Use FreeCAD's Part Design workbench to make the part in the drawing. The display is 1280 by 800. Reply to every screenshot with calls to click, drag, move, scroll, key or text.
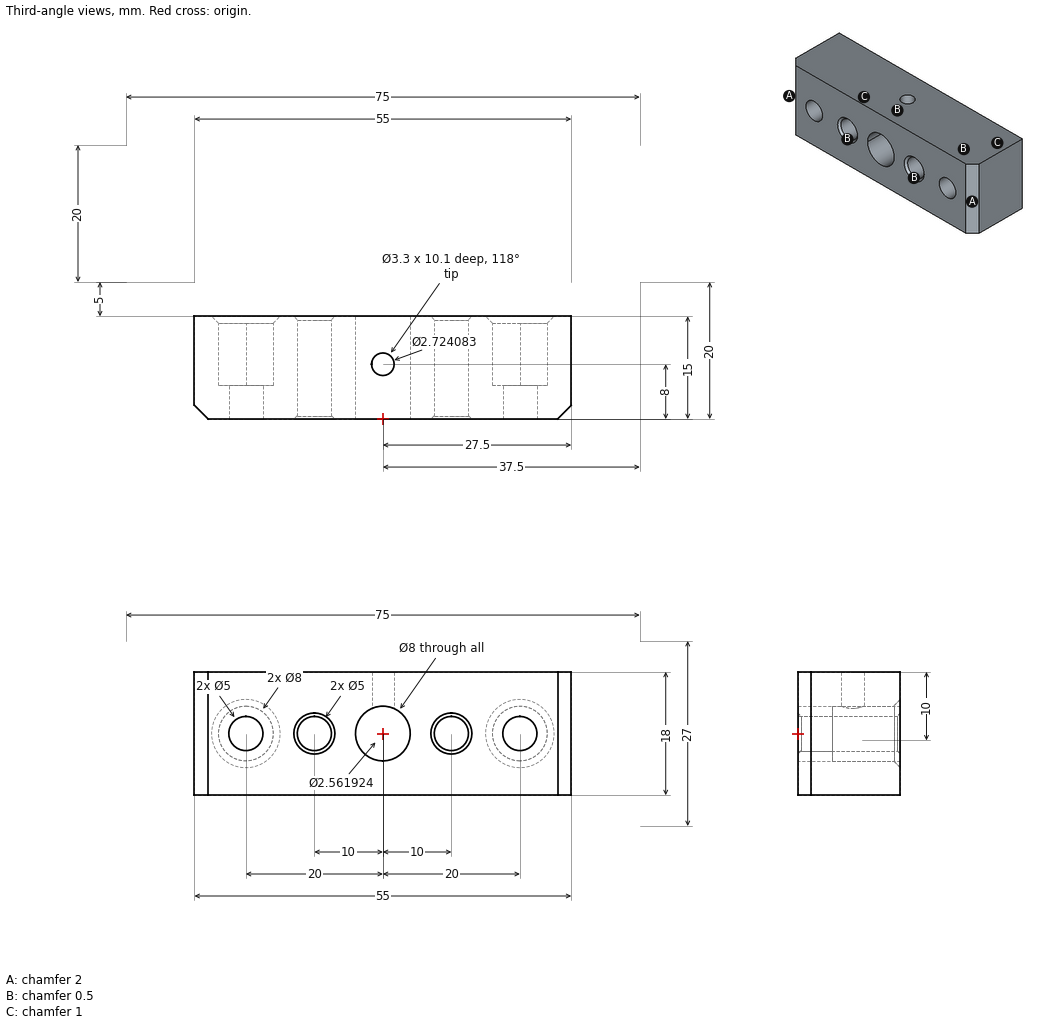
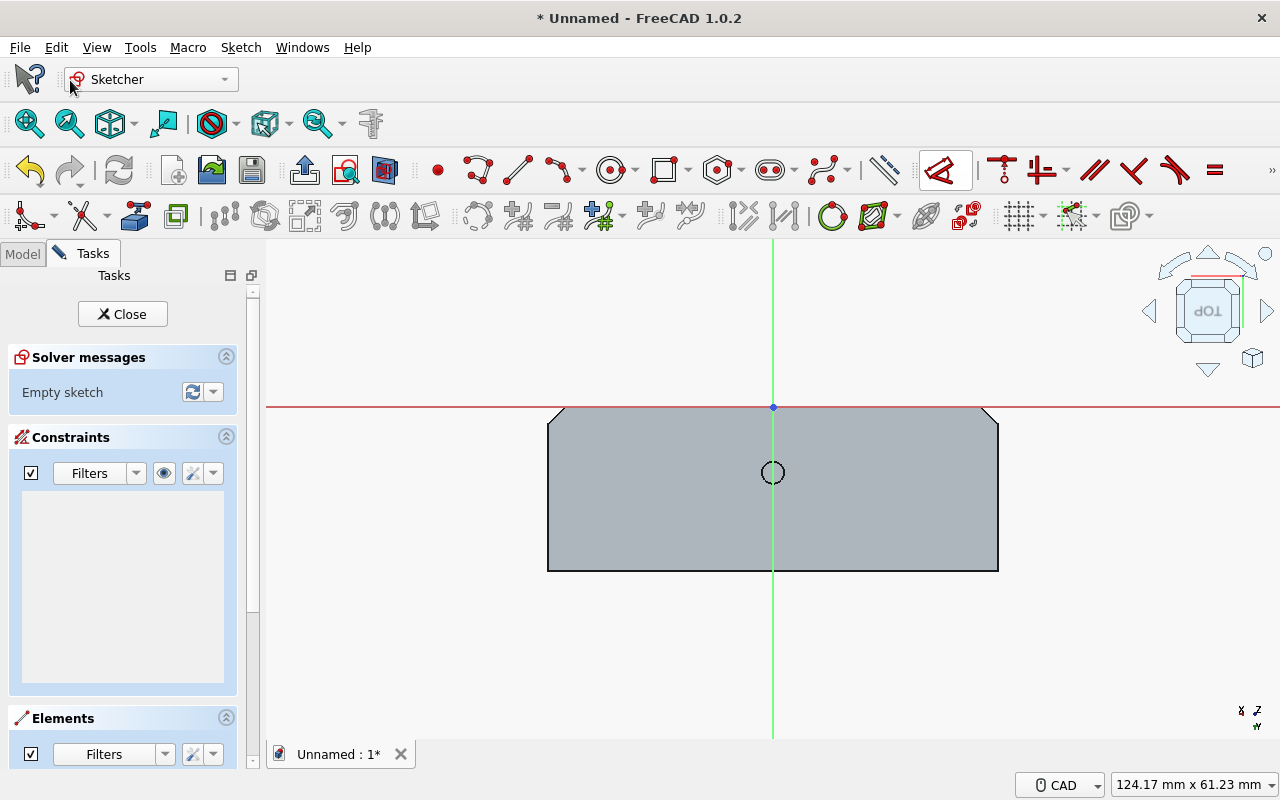
scroll(780, 471, up, 12)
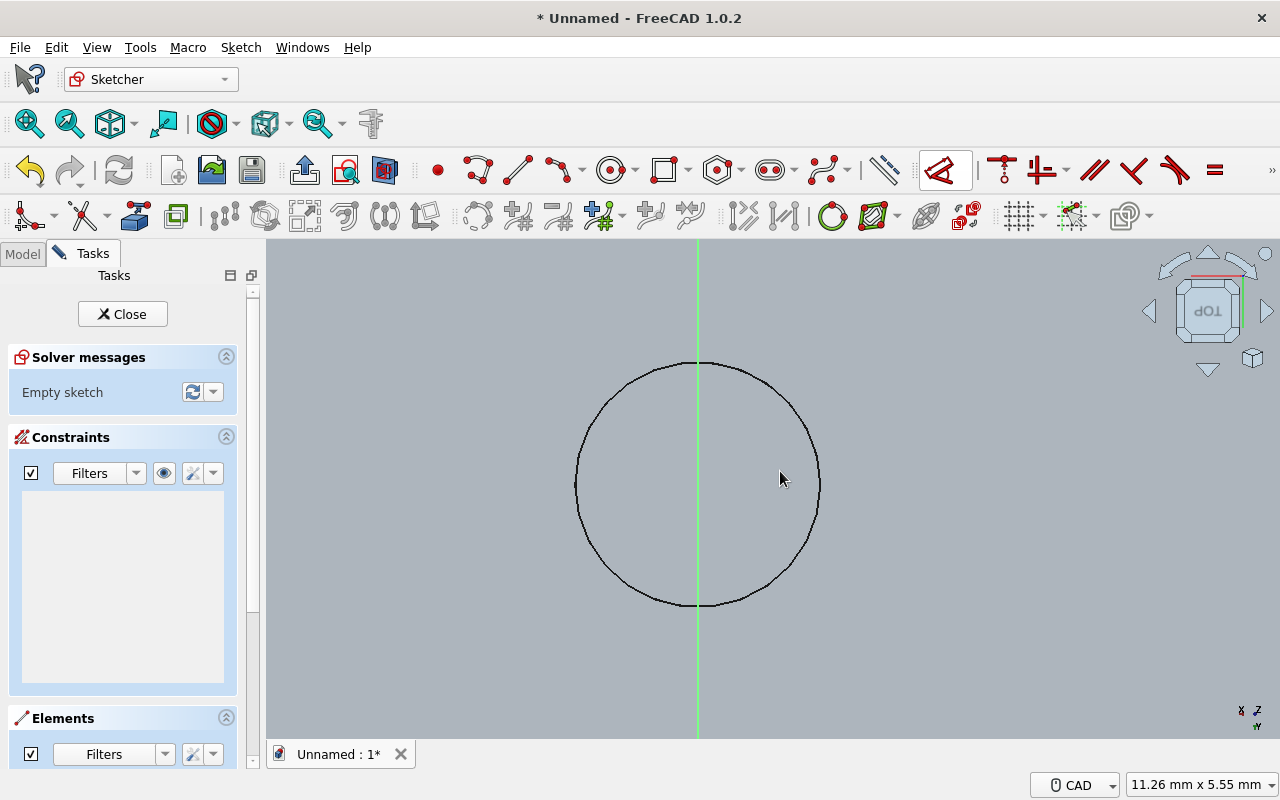
click(612, 170)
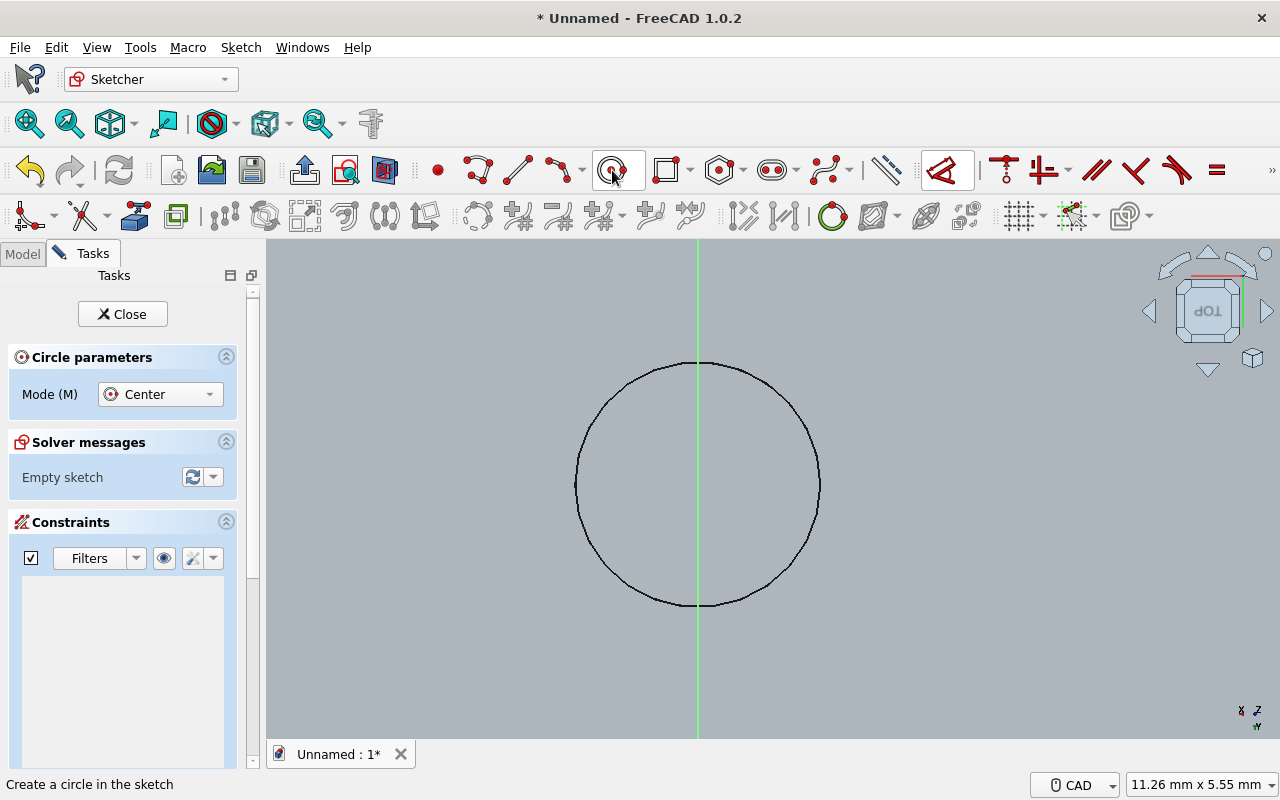
click(698, 485)
move(803, 380)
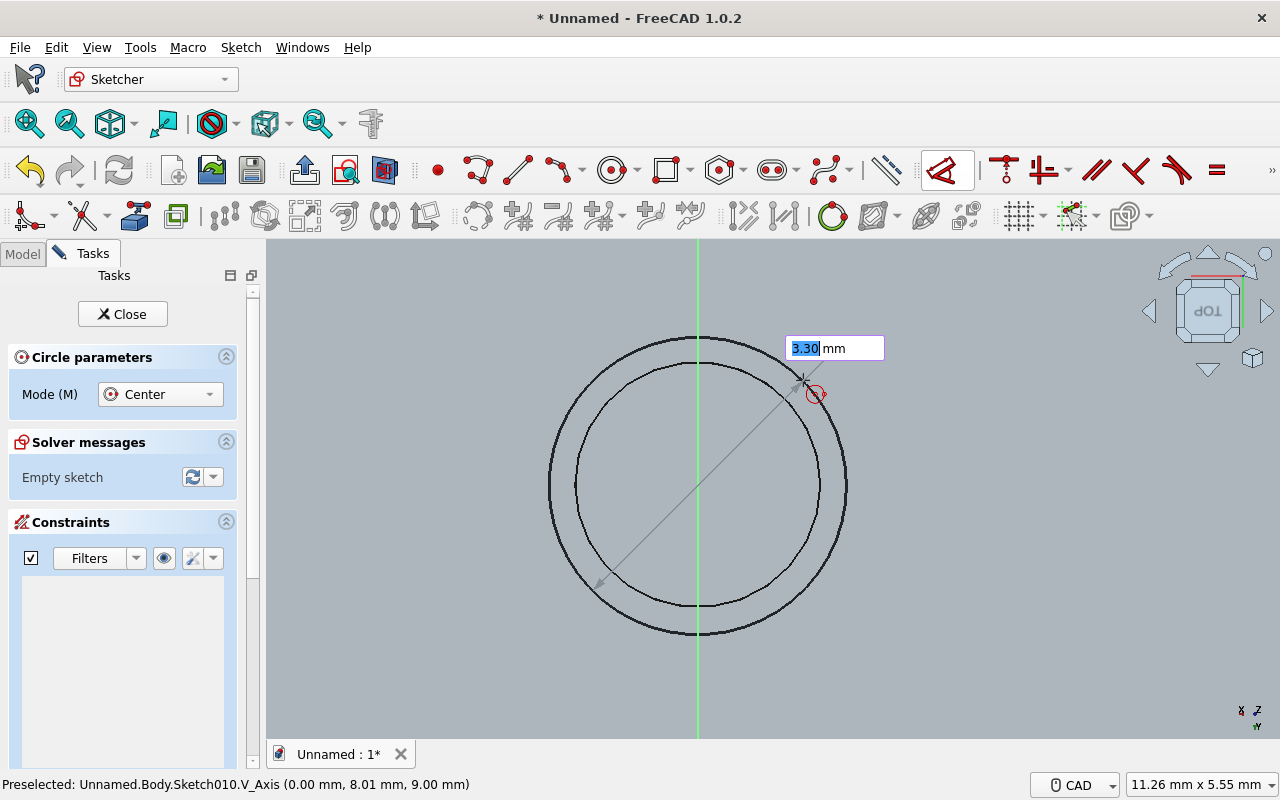
text(3.3)
key(Return)
key(Escape)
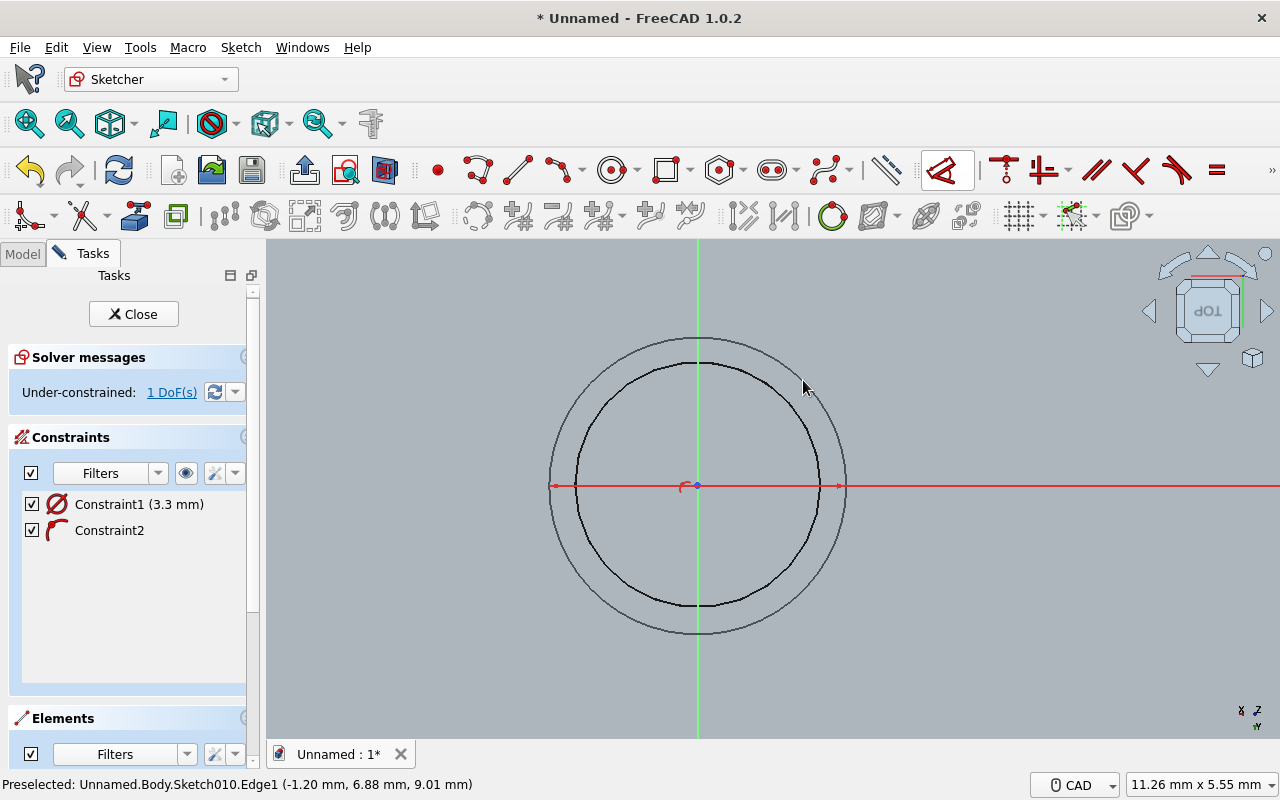
click(698, 486)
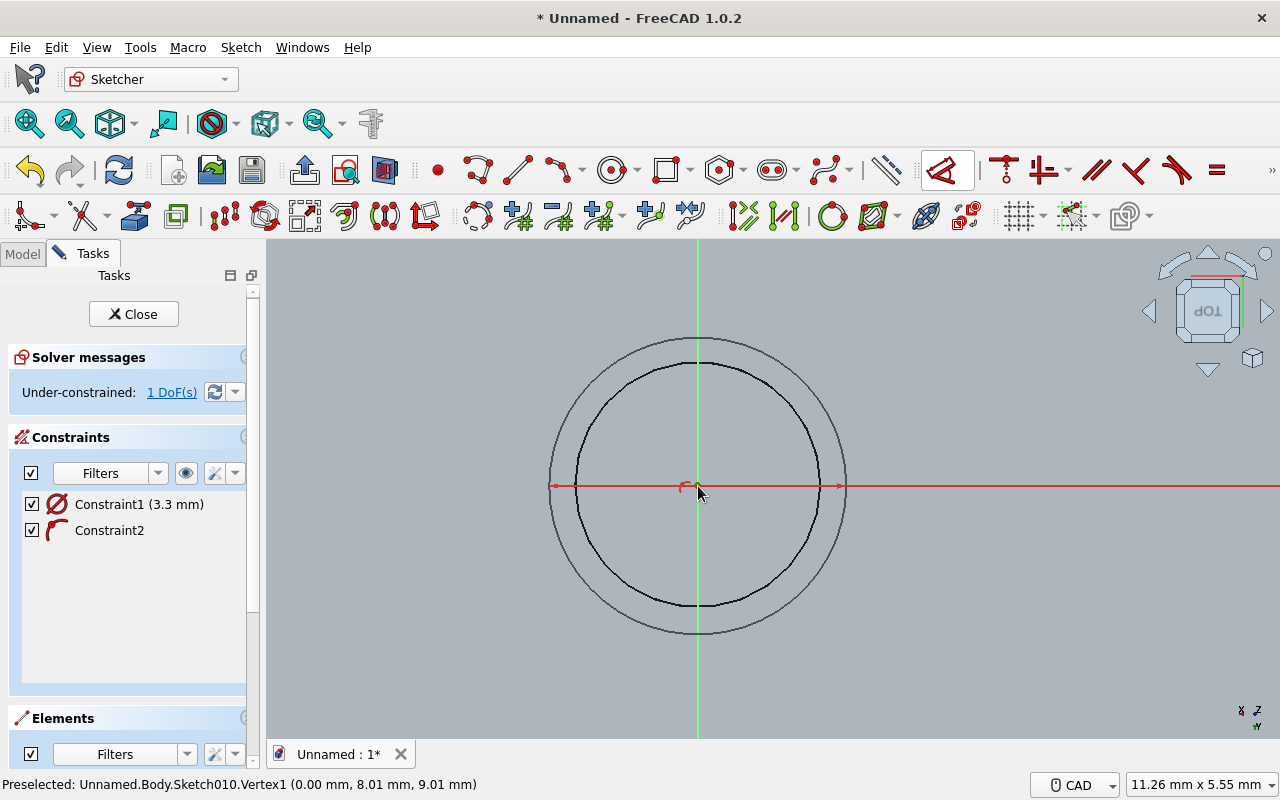
click(968, 170)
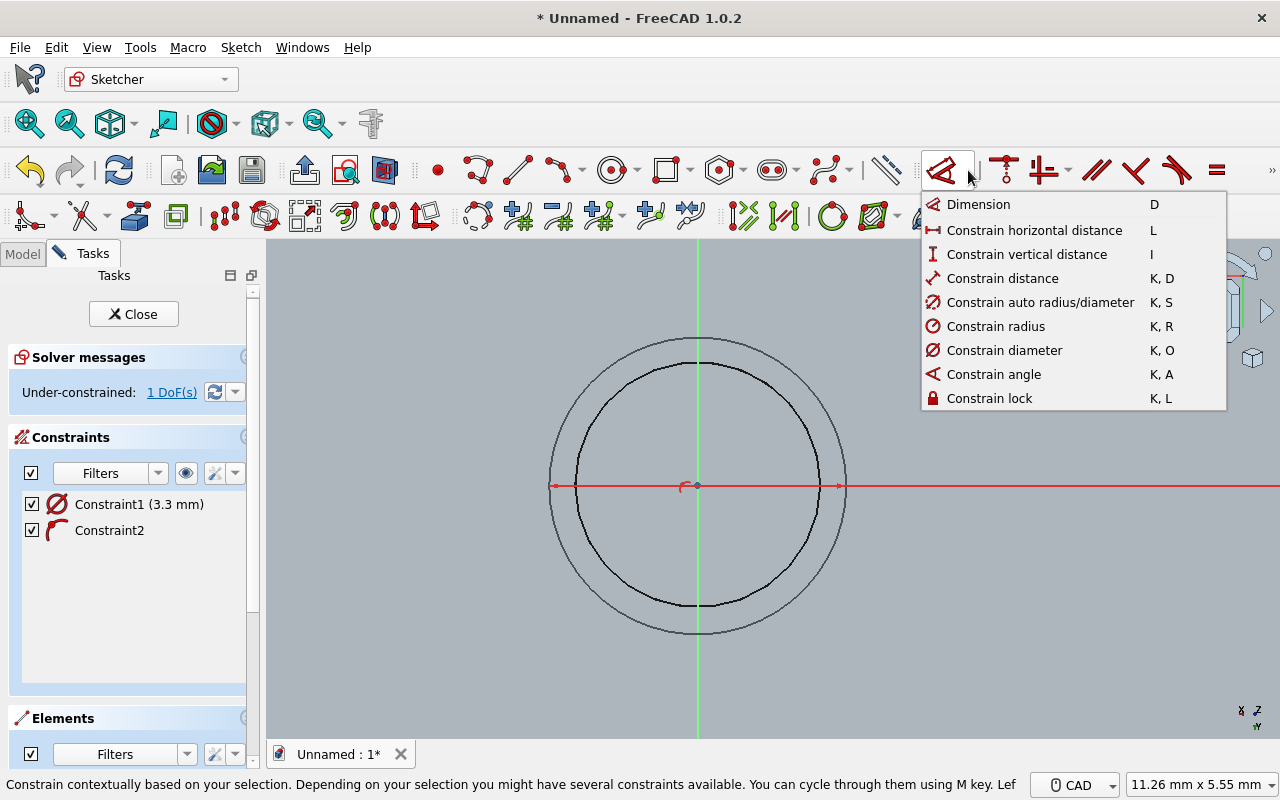
click(1074, 254)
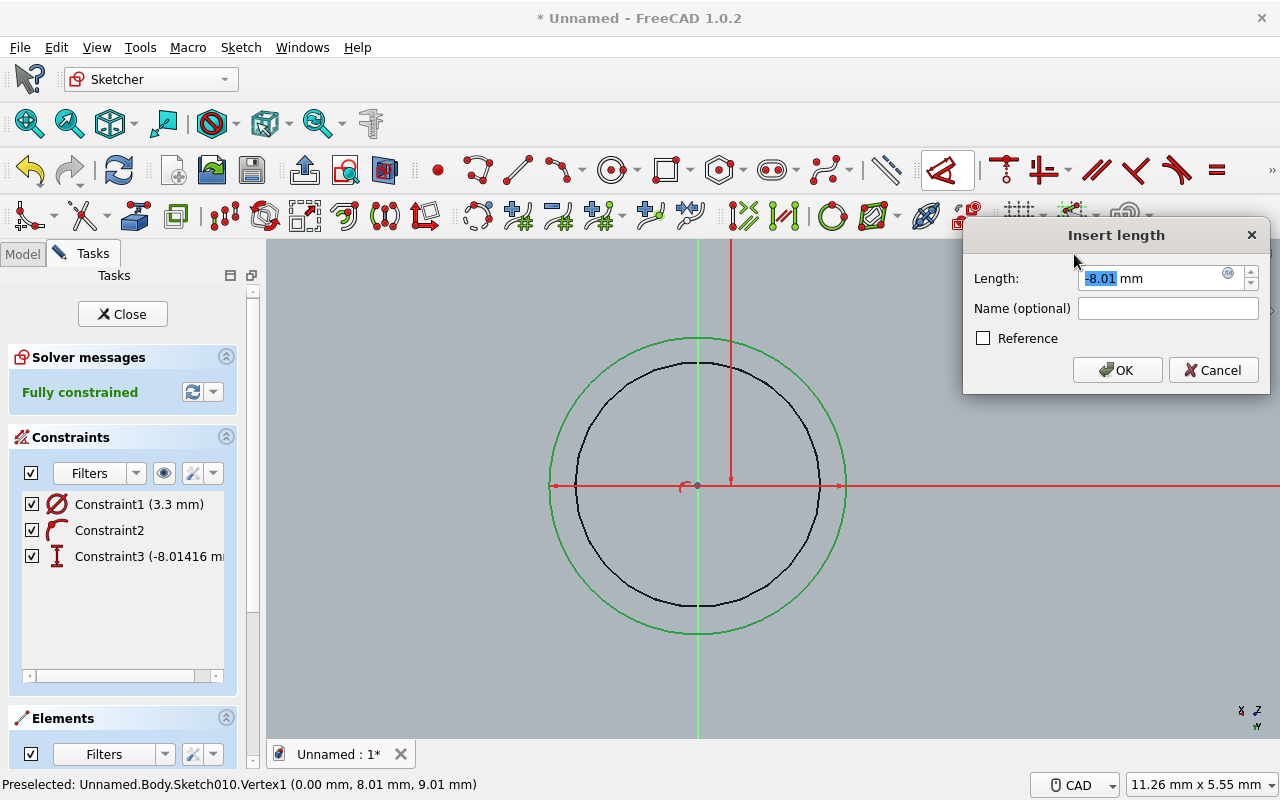
text(-8)
key(Return)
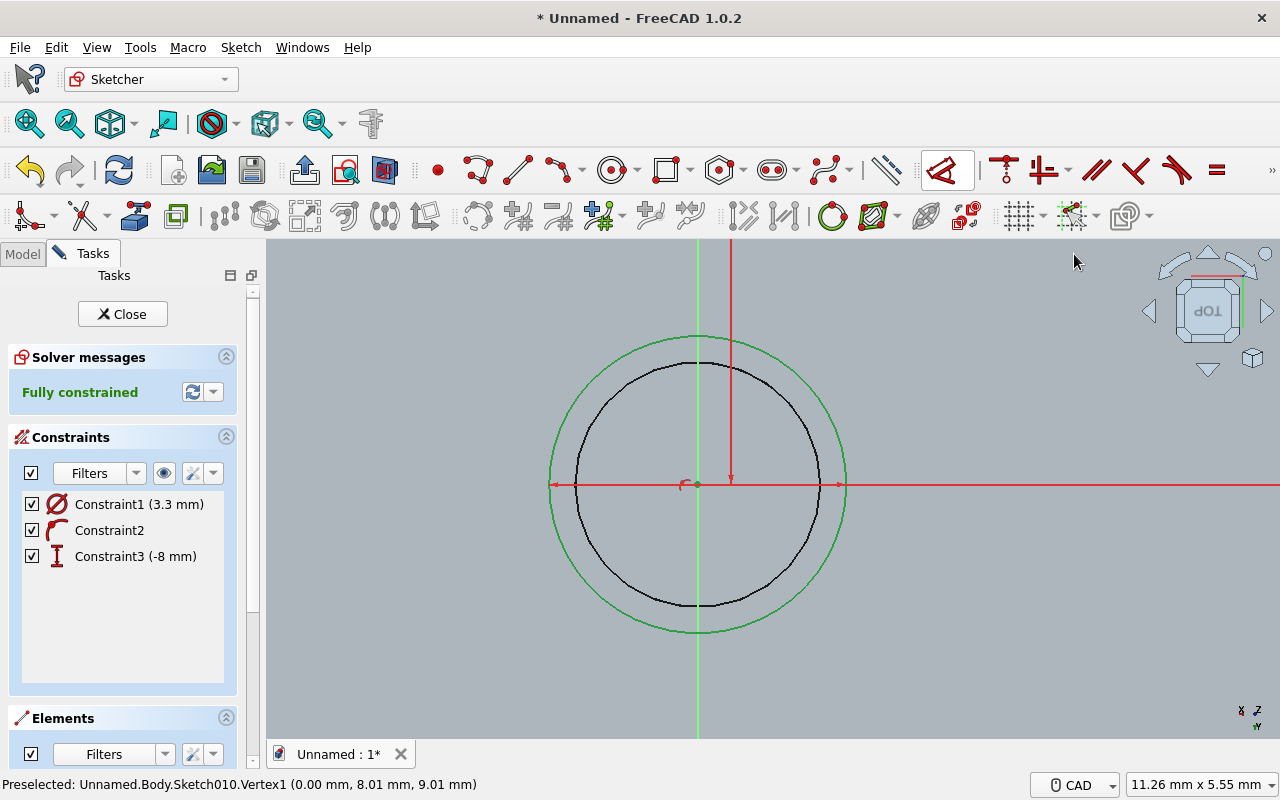
click(123, 314)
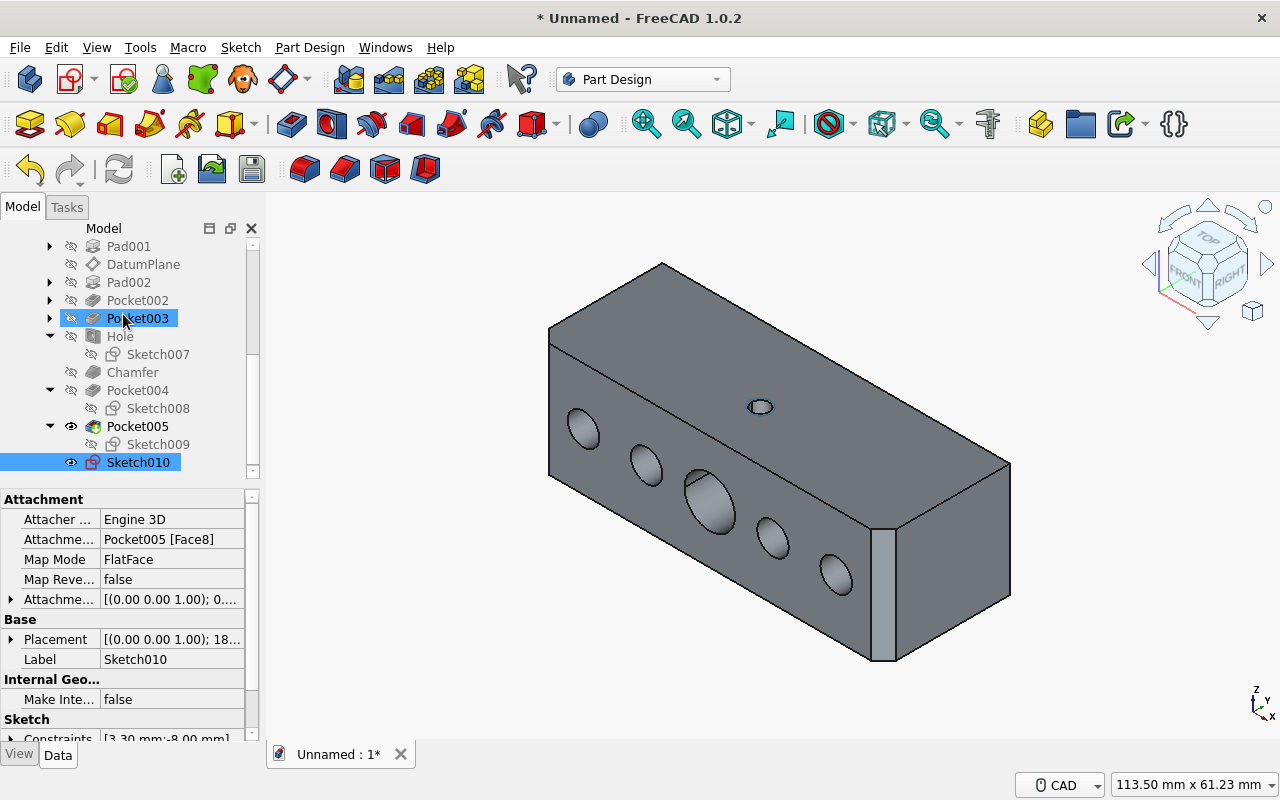
click(332, 124)